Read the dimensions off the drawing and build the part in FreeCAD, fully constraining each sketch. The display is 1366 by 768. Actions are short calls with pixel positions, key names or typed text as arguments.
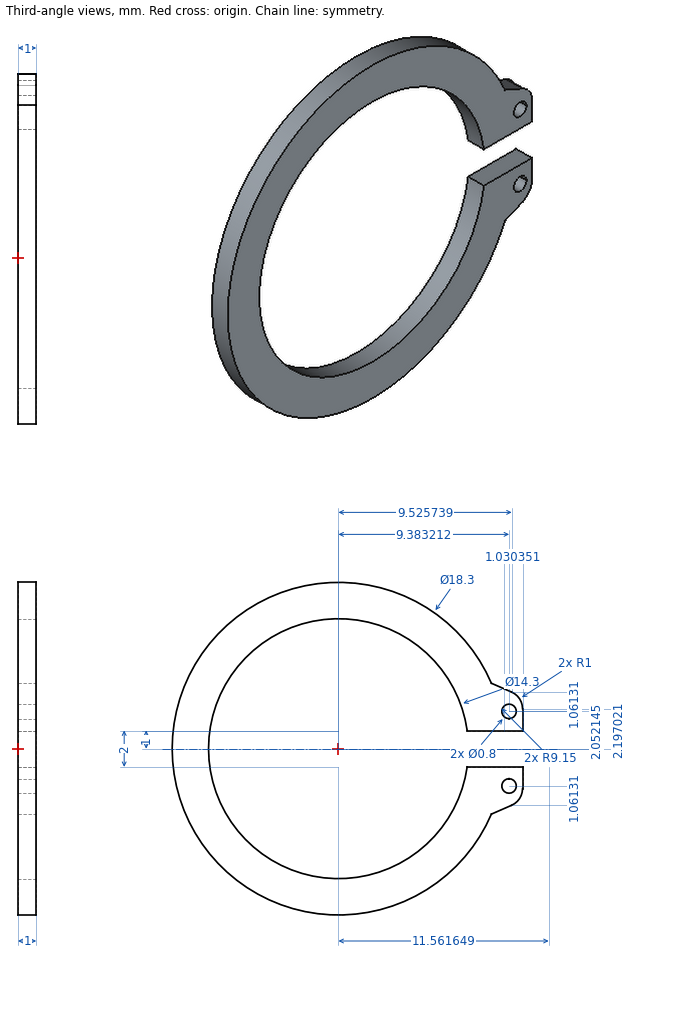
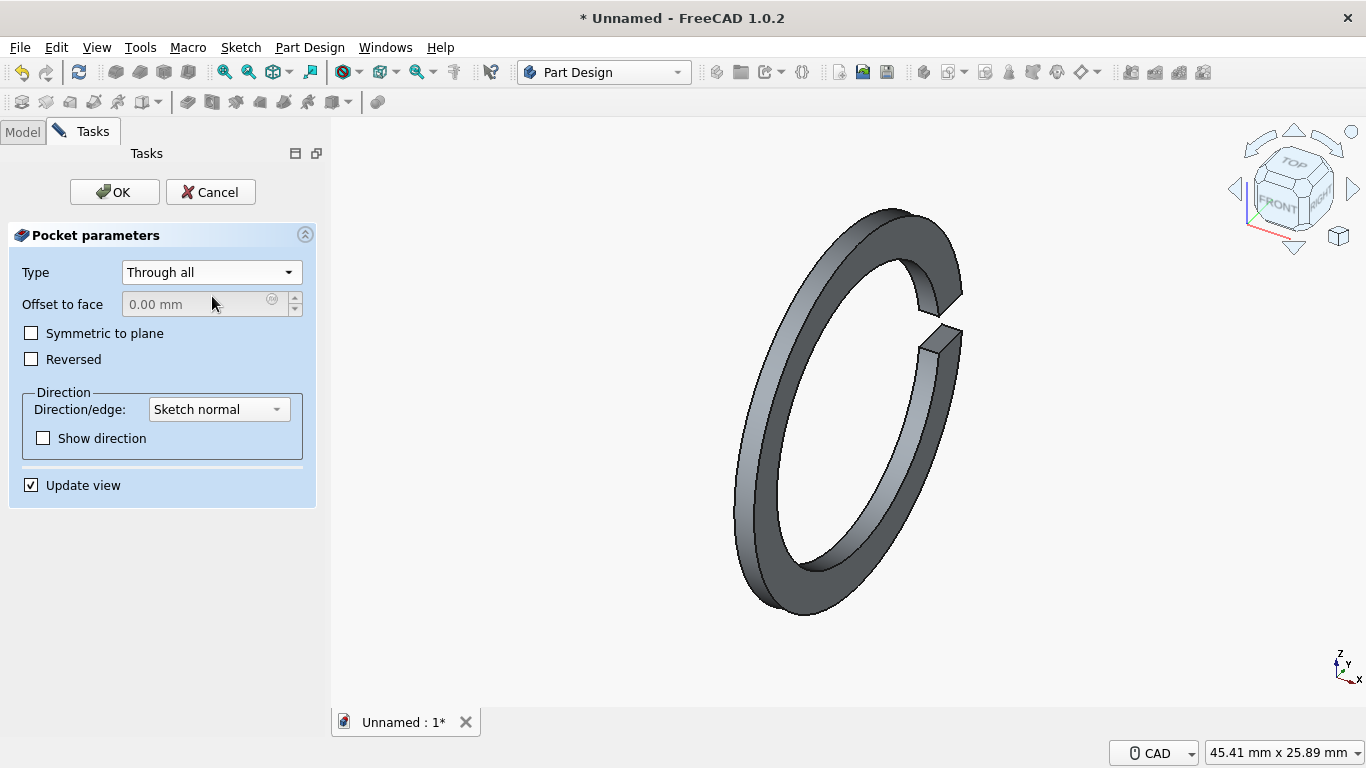
click(115, 192)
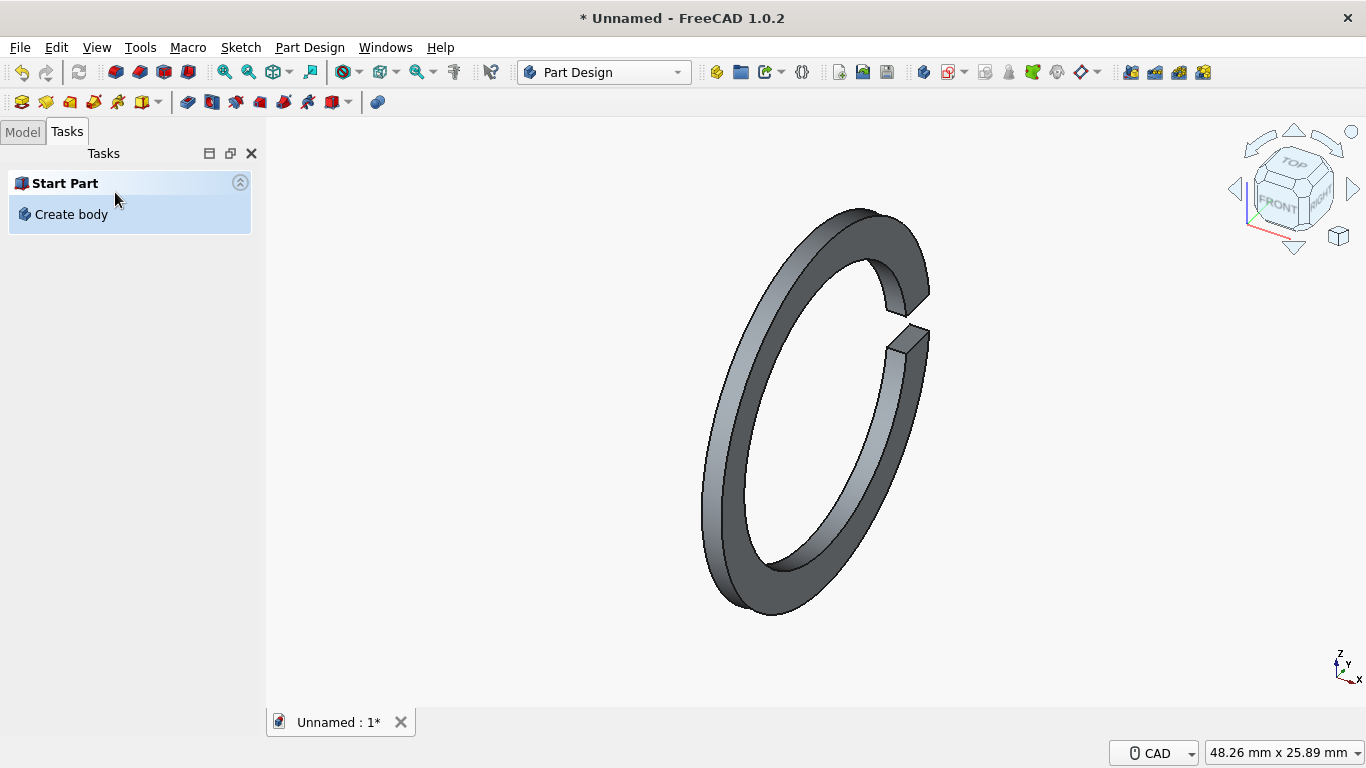
click(948, 72)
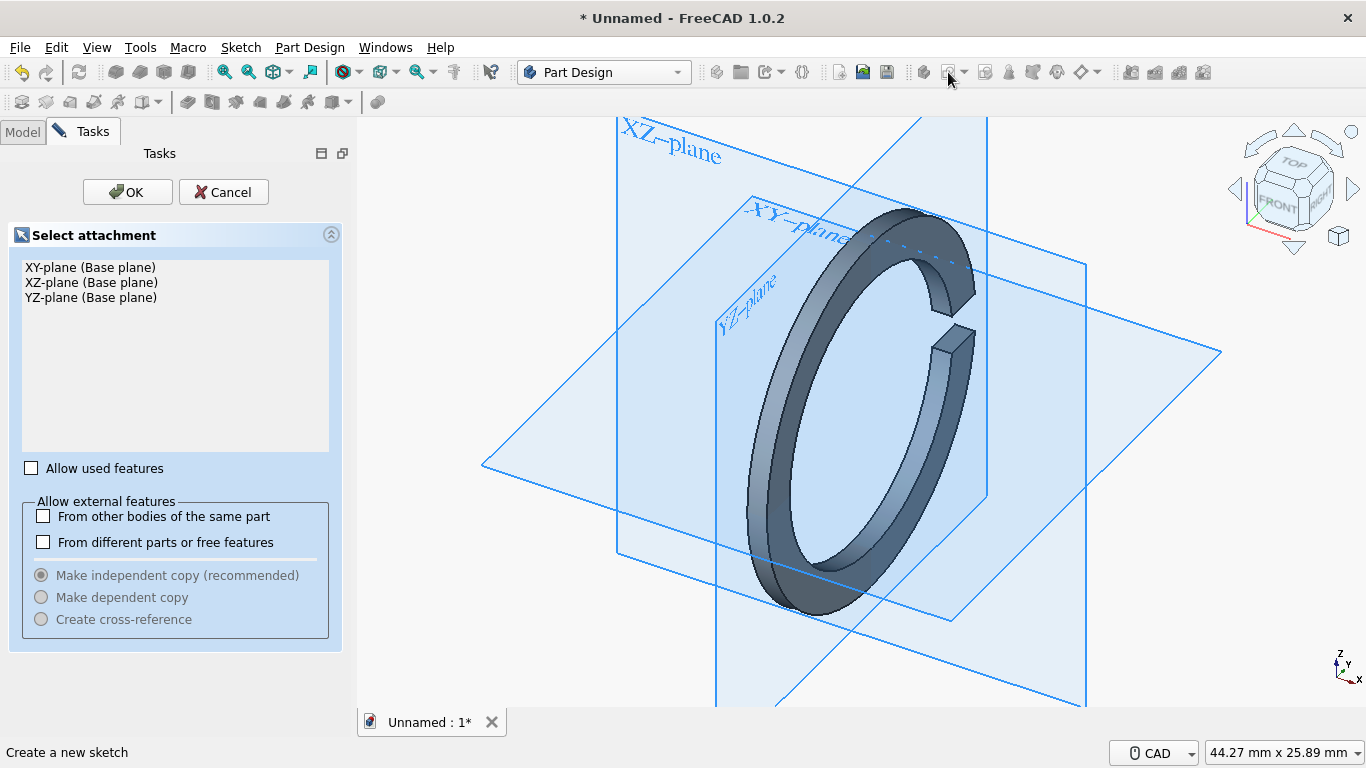
click(82, 298)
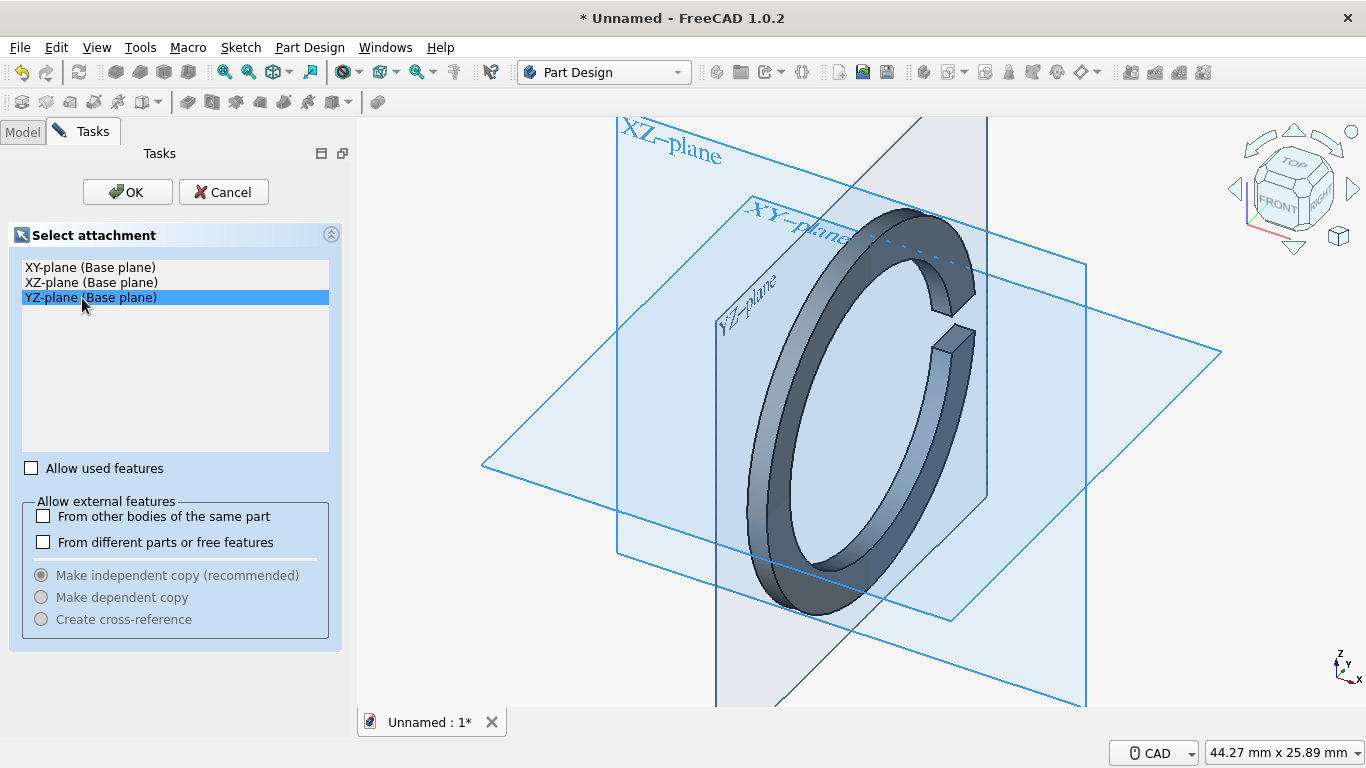
click(128, 192)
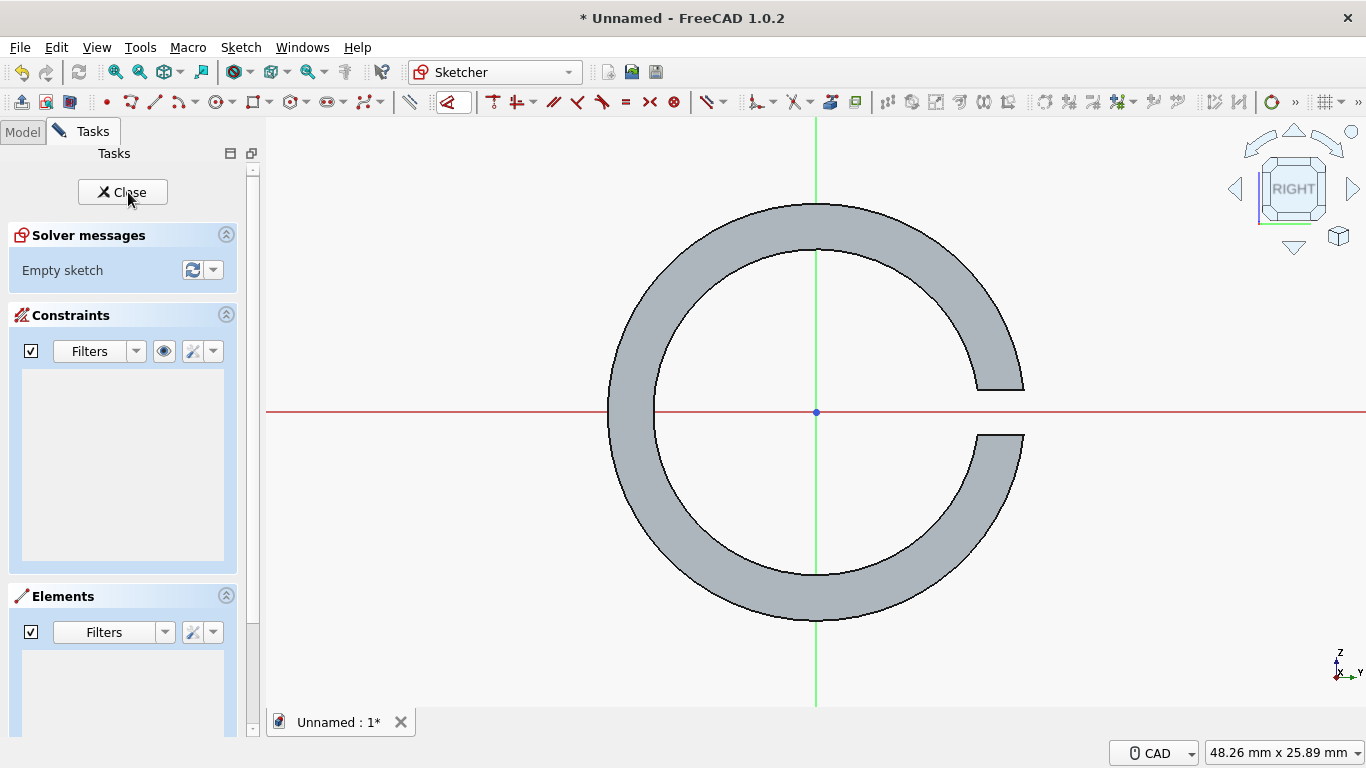
click(70, 102)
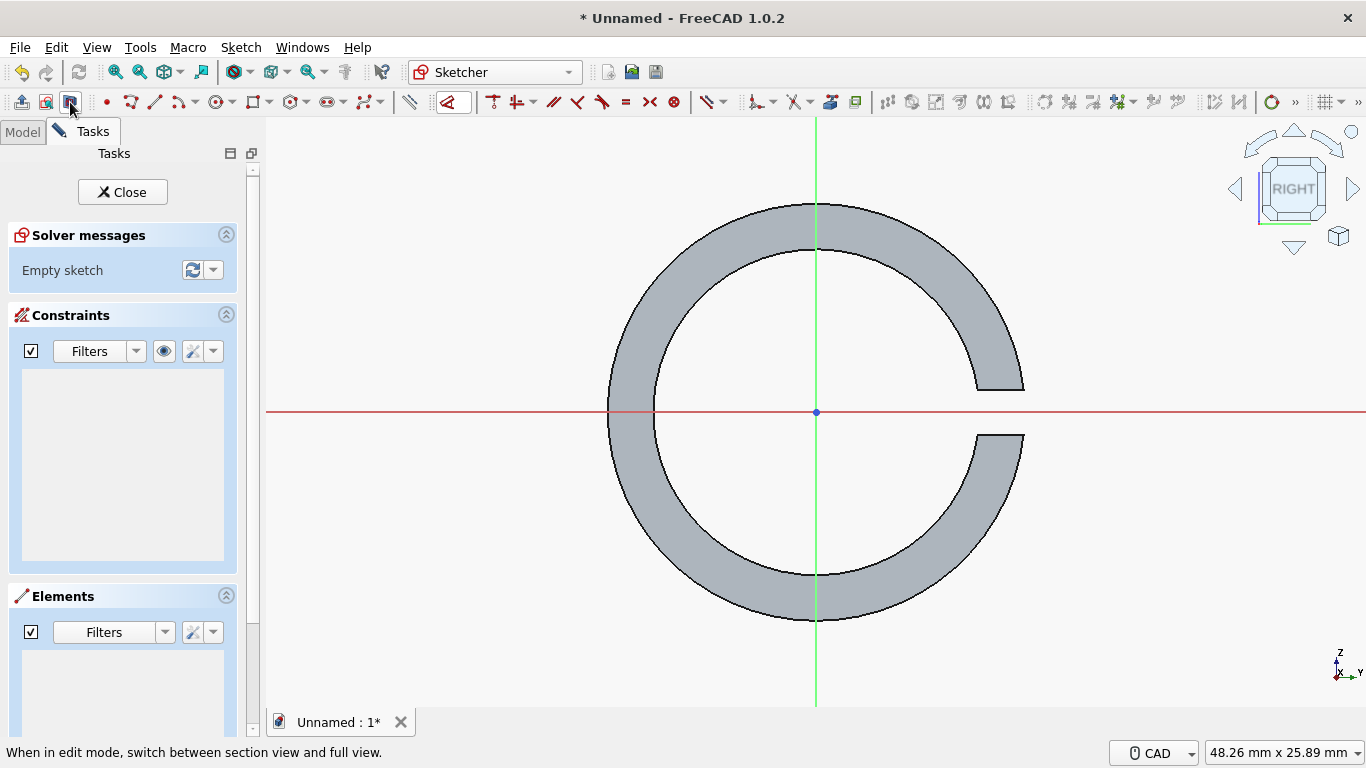
scroll(1082, 413, up, 4)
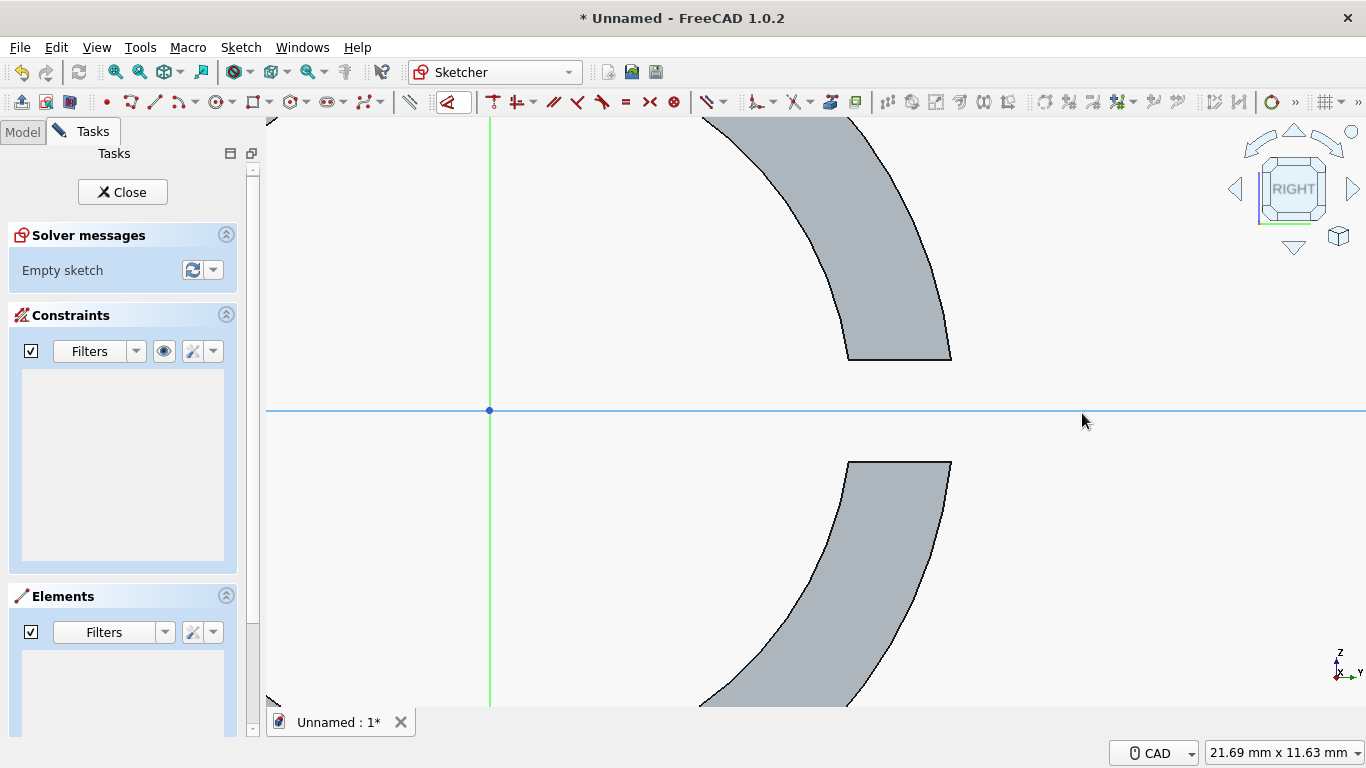
click(132, 102)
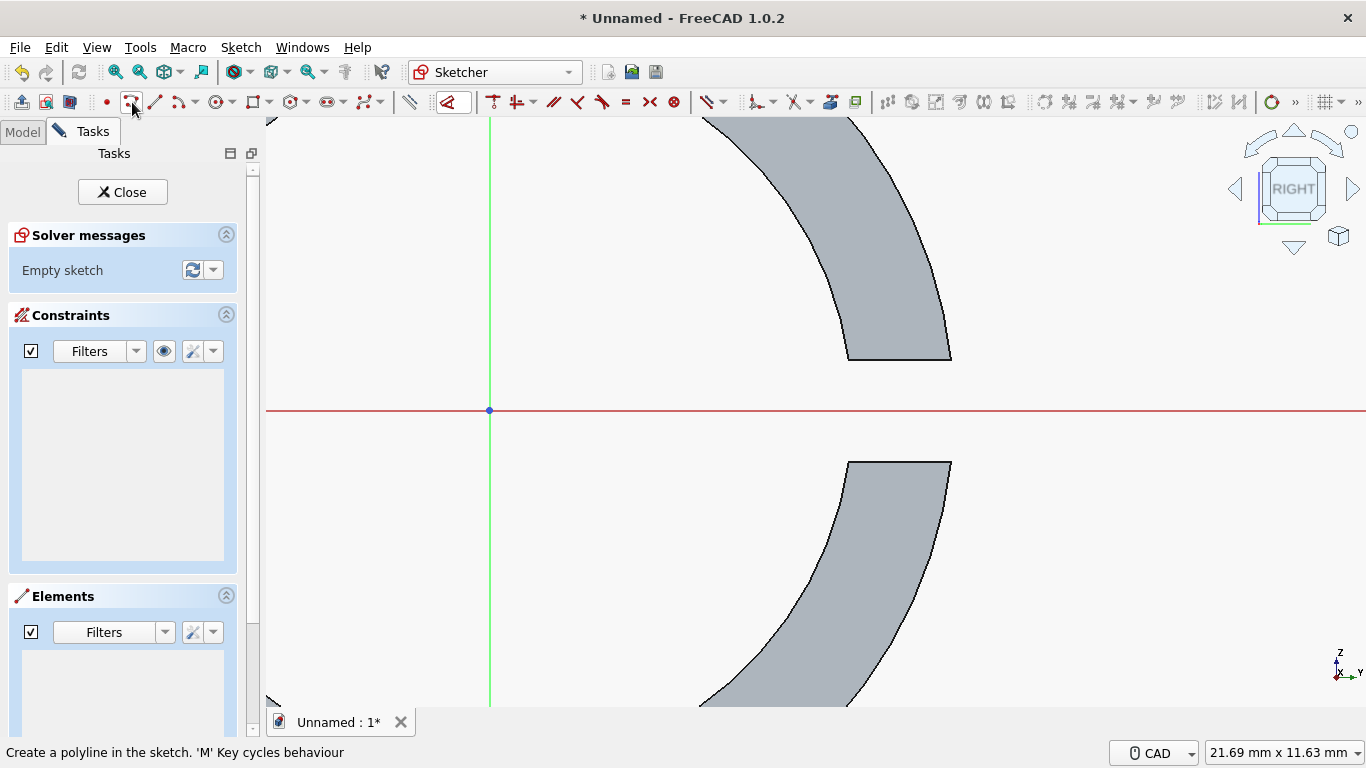
click(951, 360)
click(1003, 360)
click(1007, 299)
right_click(1007, 299)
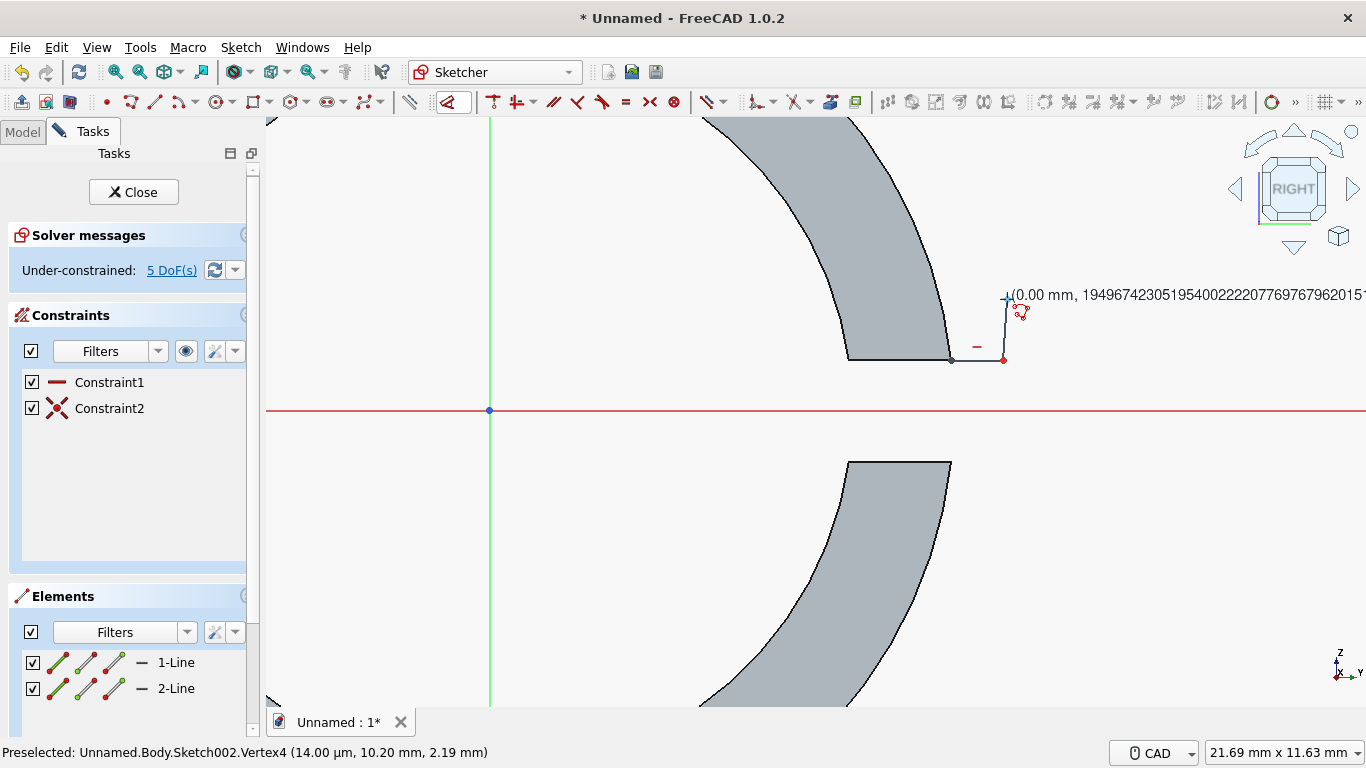
click(156, 102)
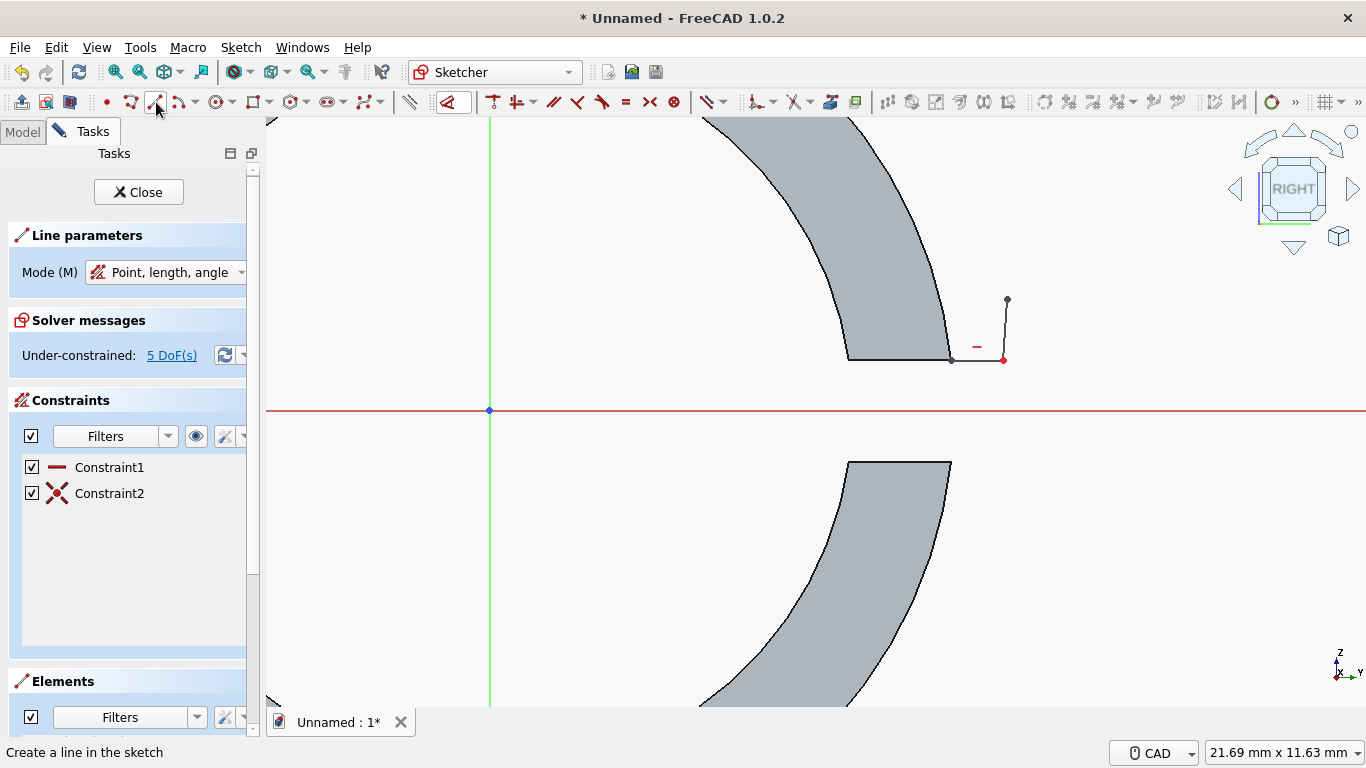
click(973, 253)
click(916, 228)